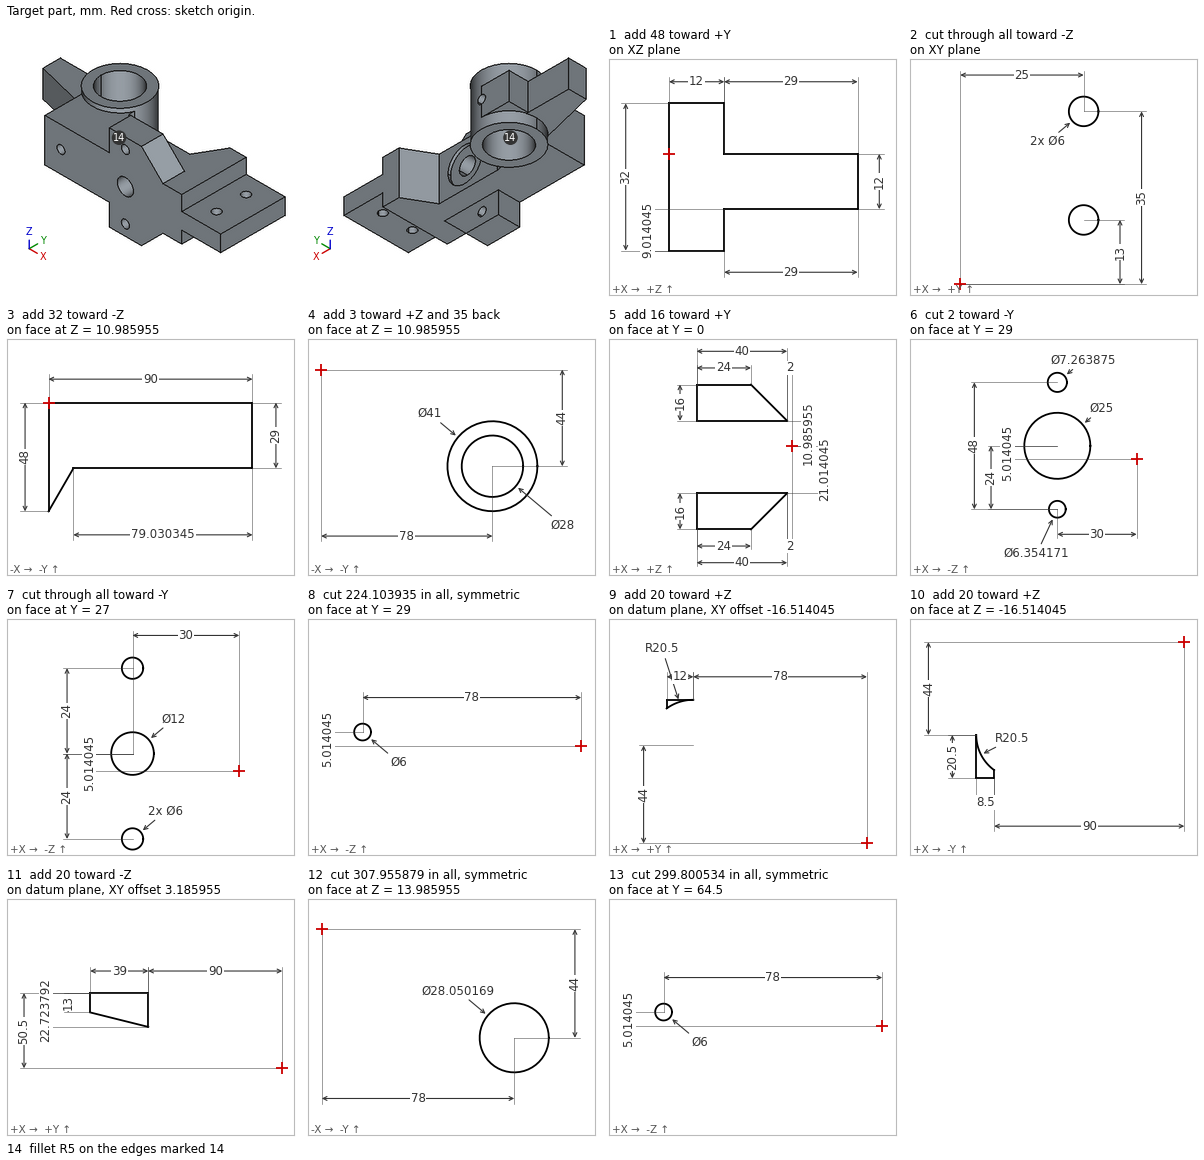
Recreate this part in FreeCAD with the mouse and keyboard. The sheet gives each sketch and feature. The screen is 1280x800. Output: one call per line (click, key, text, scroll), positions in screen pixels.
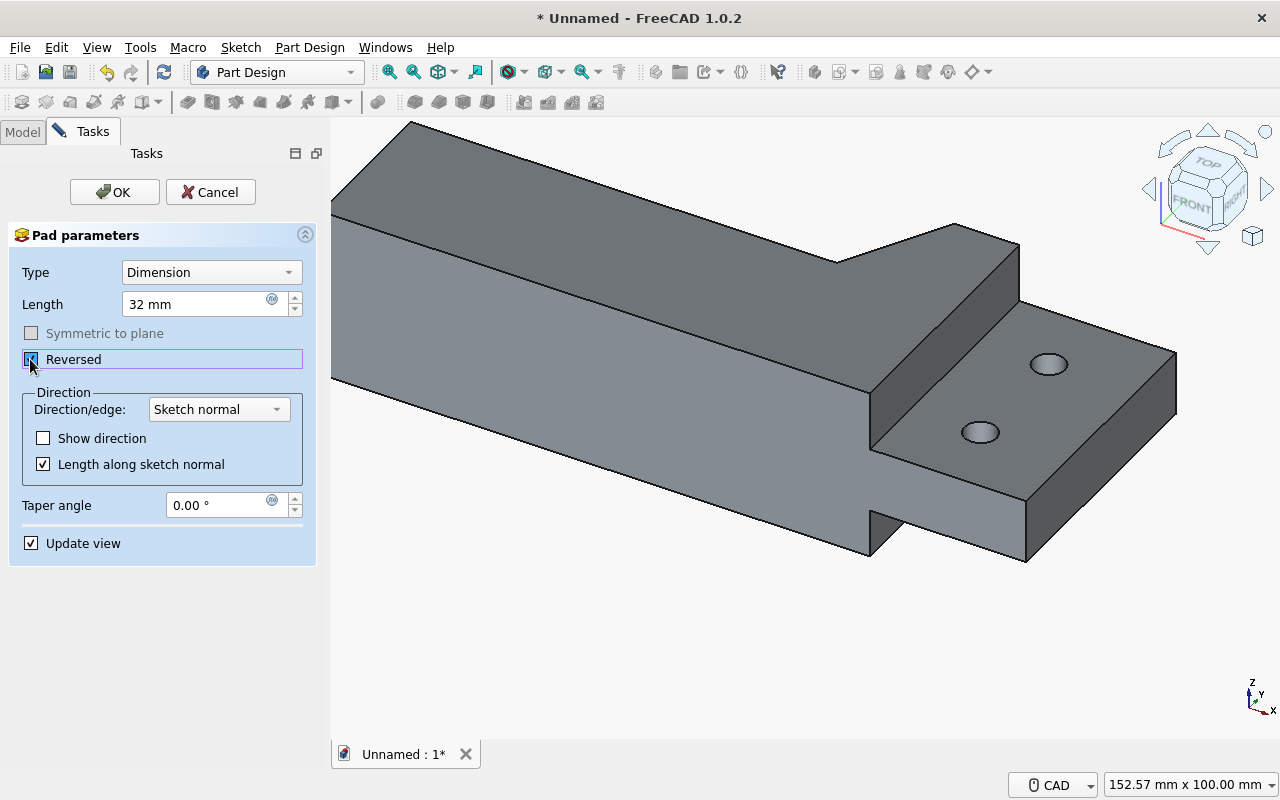
click(115, 192)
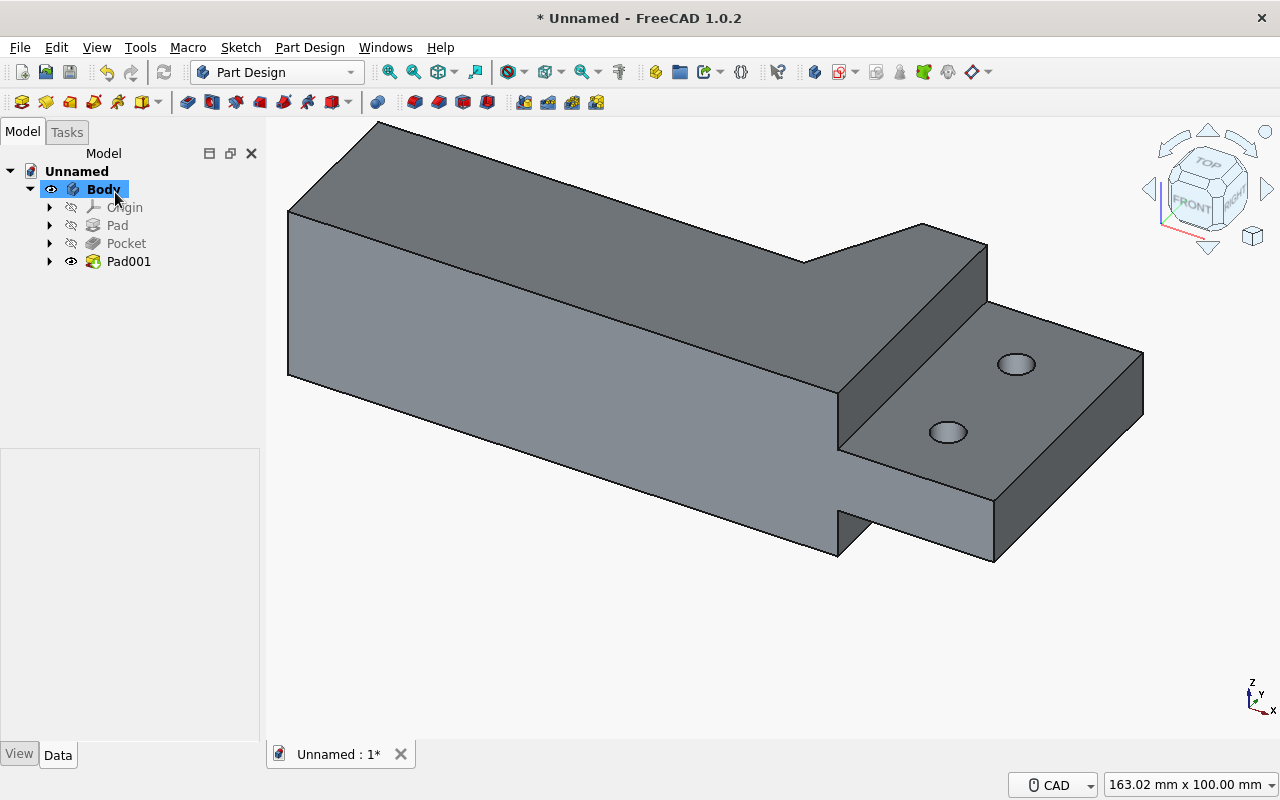
key(v)
key(f)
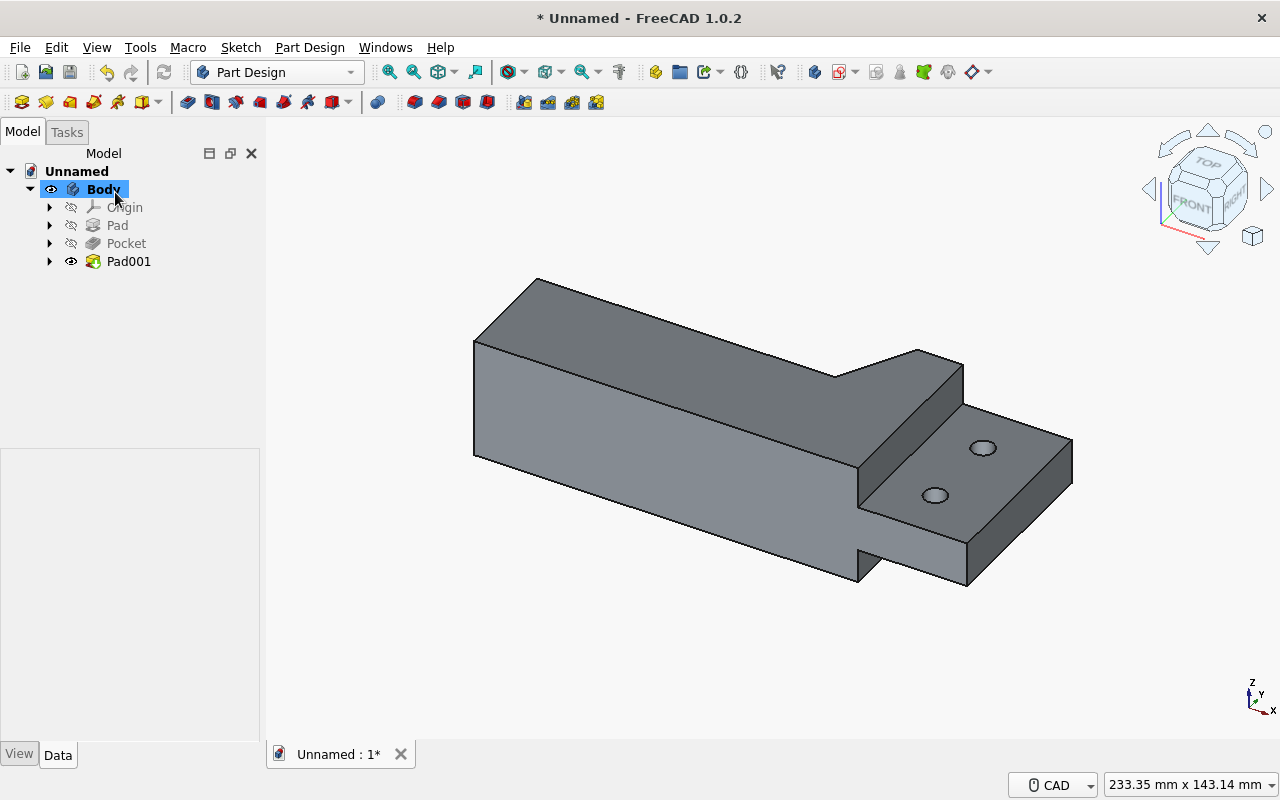
click(813, 403)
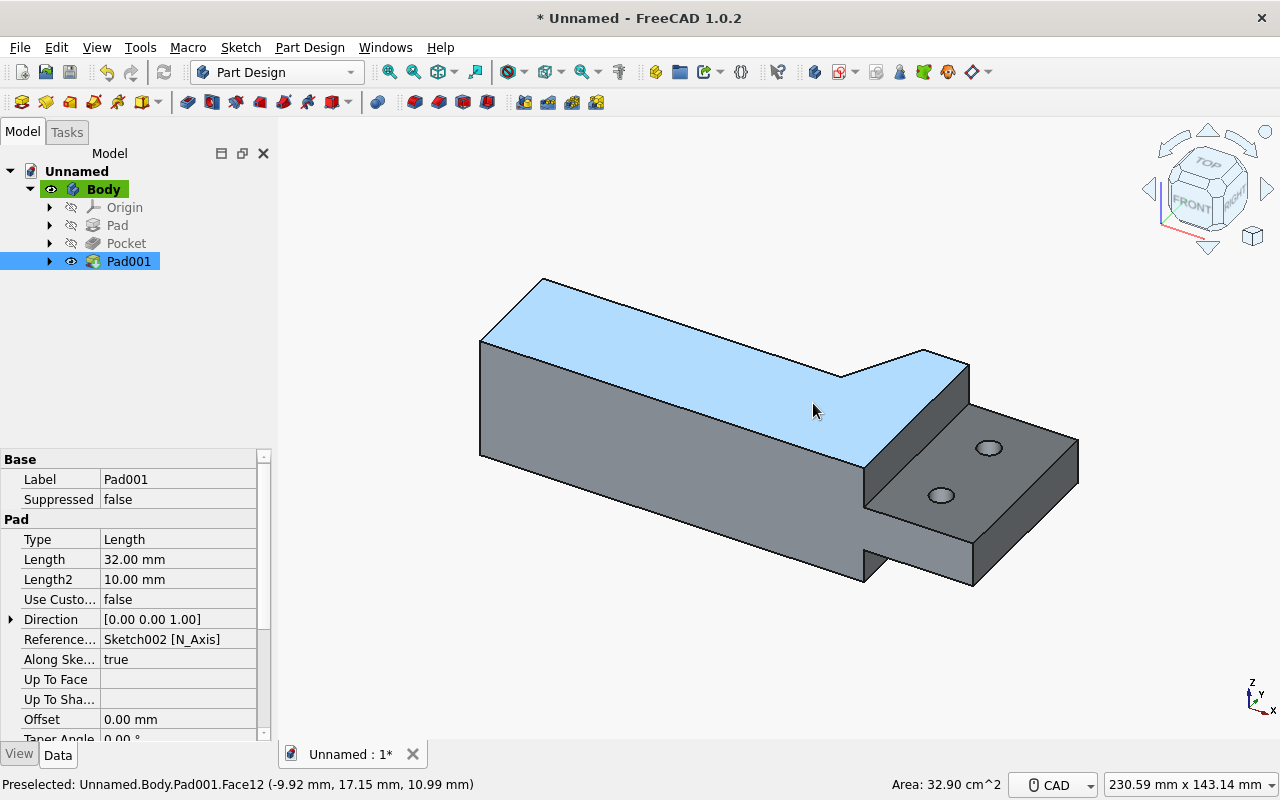
click(840, 72)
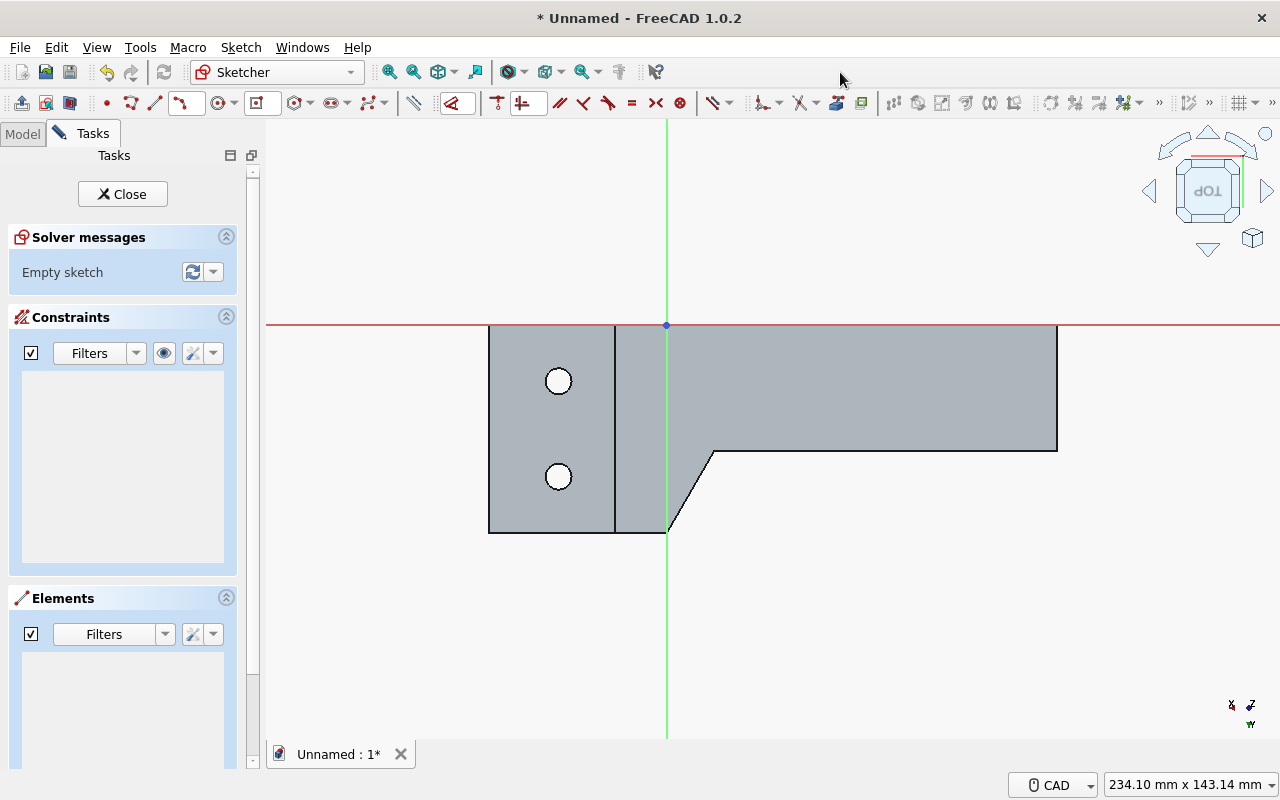
scroll(1115, 537, up, 2)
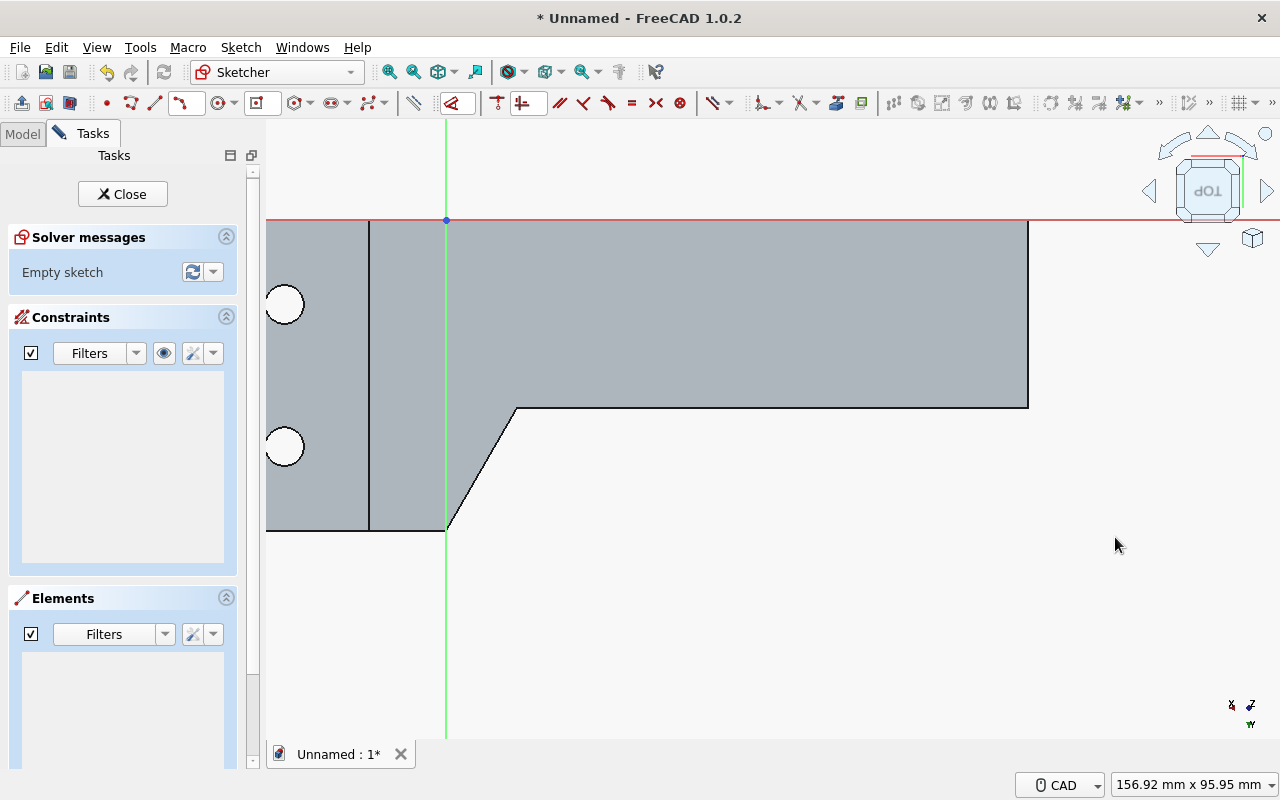
key(g)
key(c)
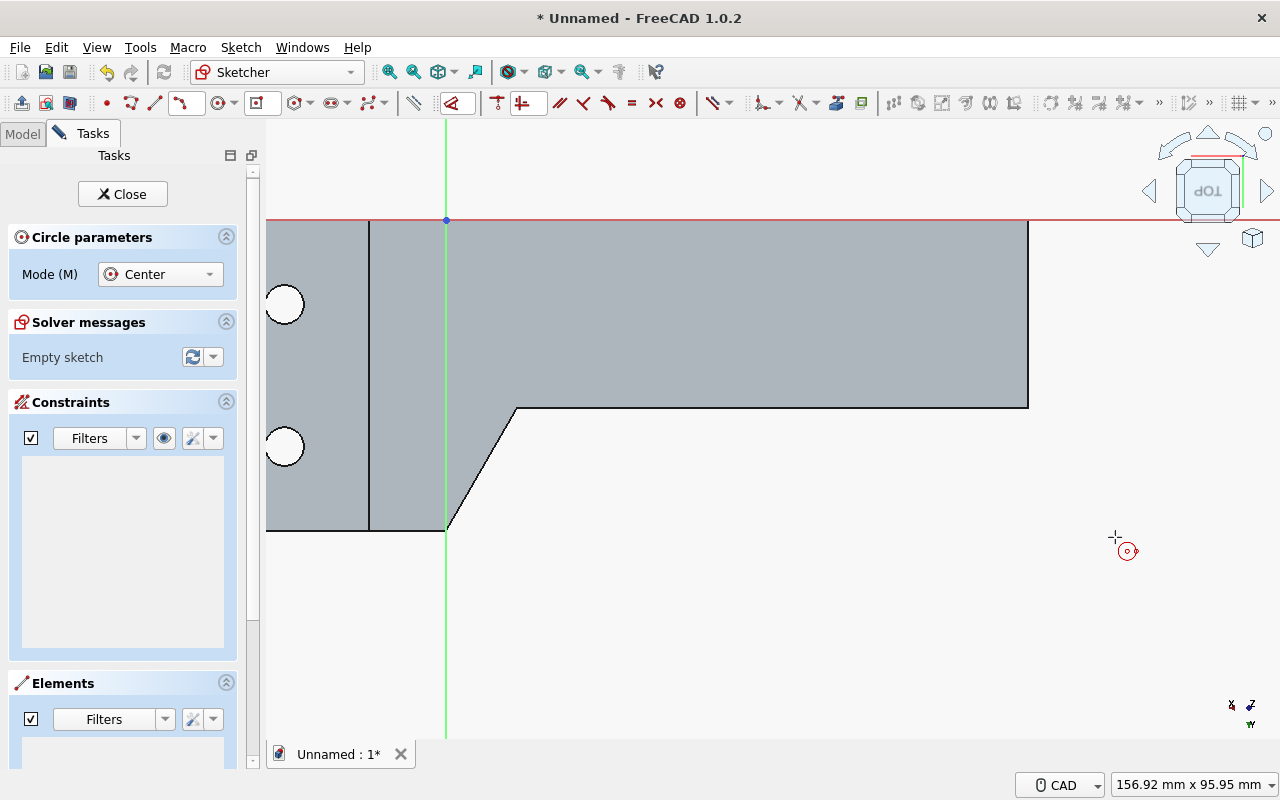
click(950, 505)
move(1044, 411)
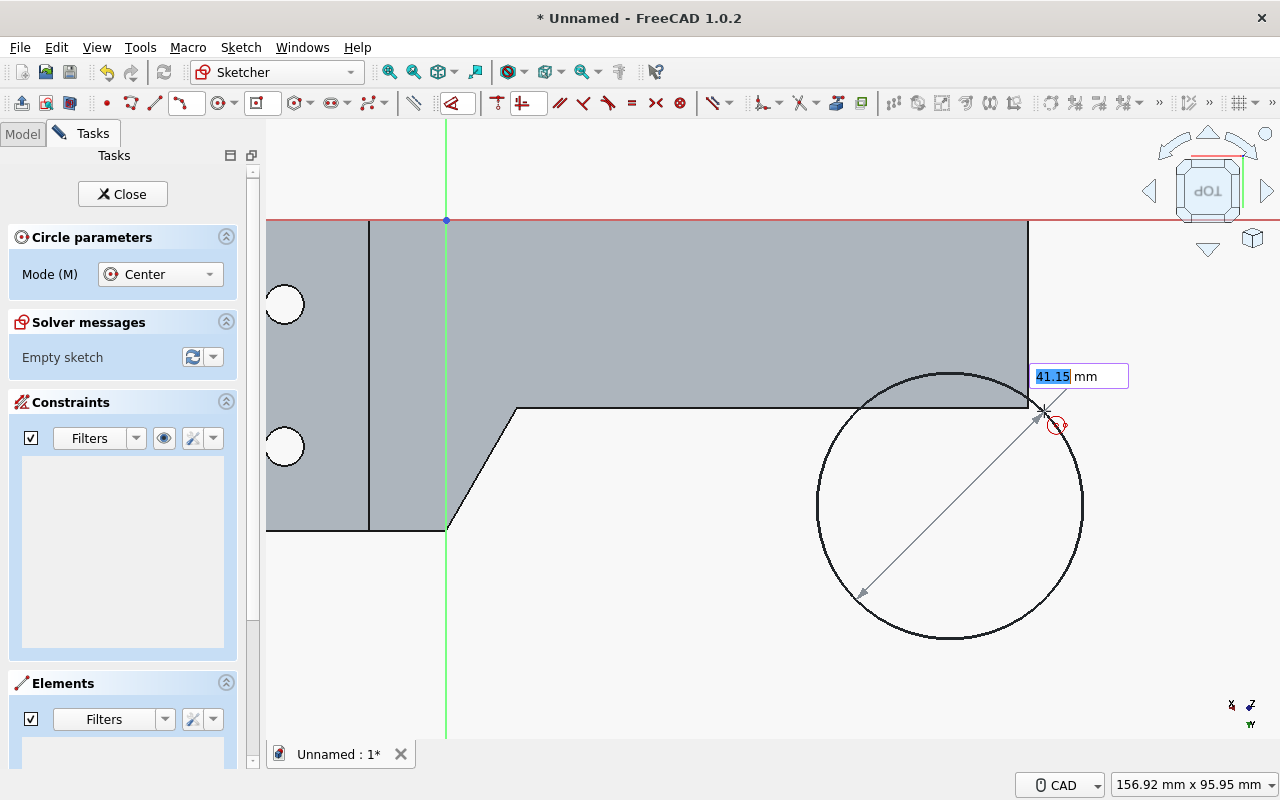
text(41)
key(Return)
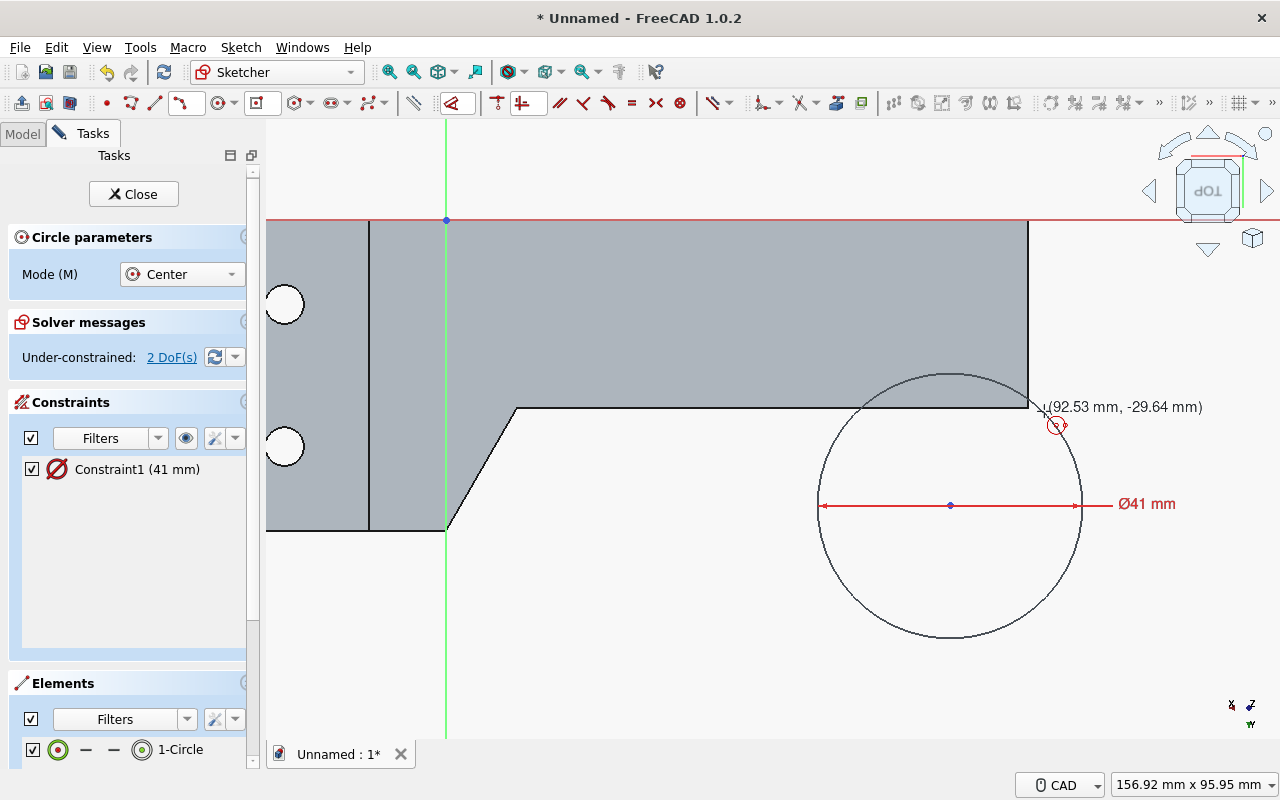
click(950, 506)
move(1014, 441)